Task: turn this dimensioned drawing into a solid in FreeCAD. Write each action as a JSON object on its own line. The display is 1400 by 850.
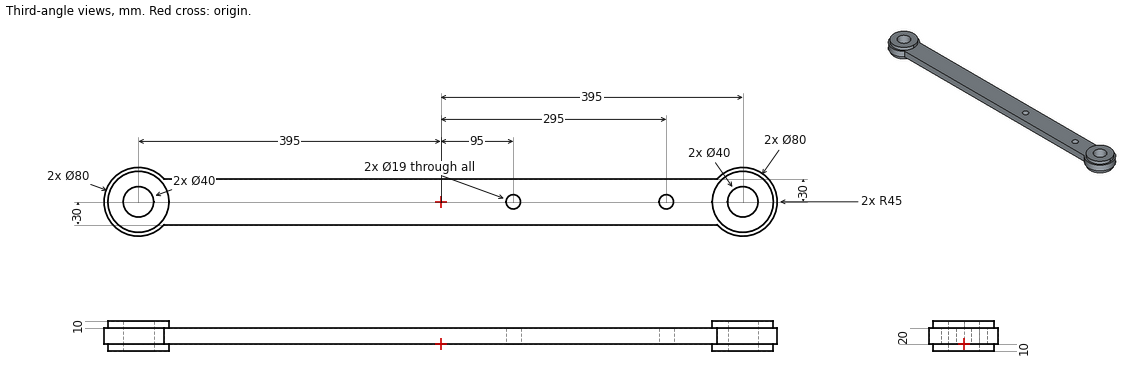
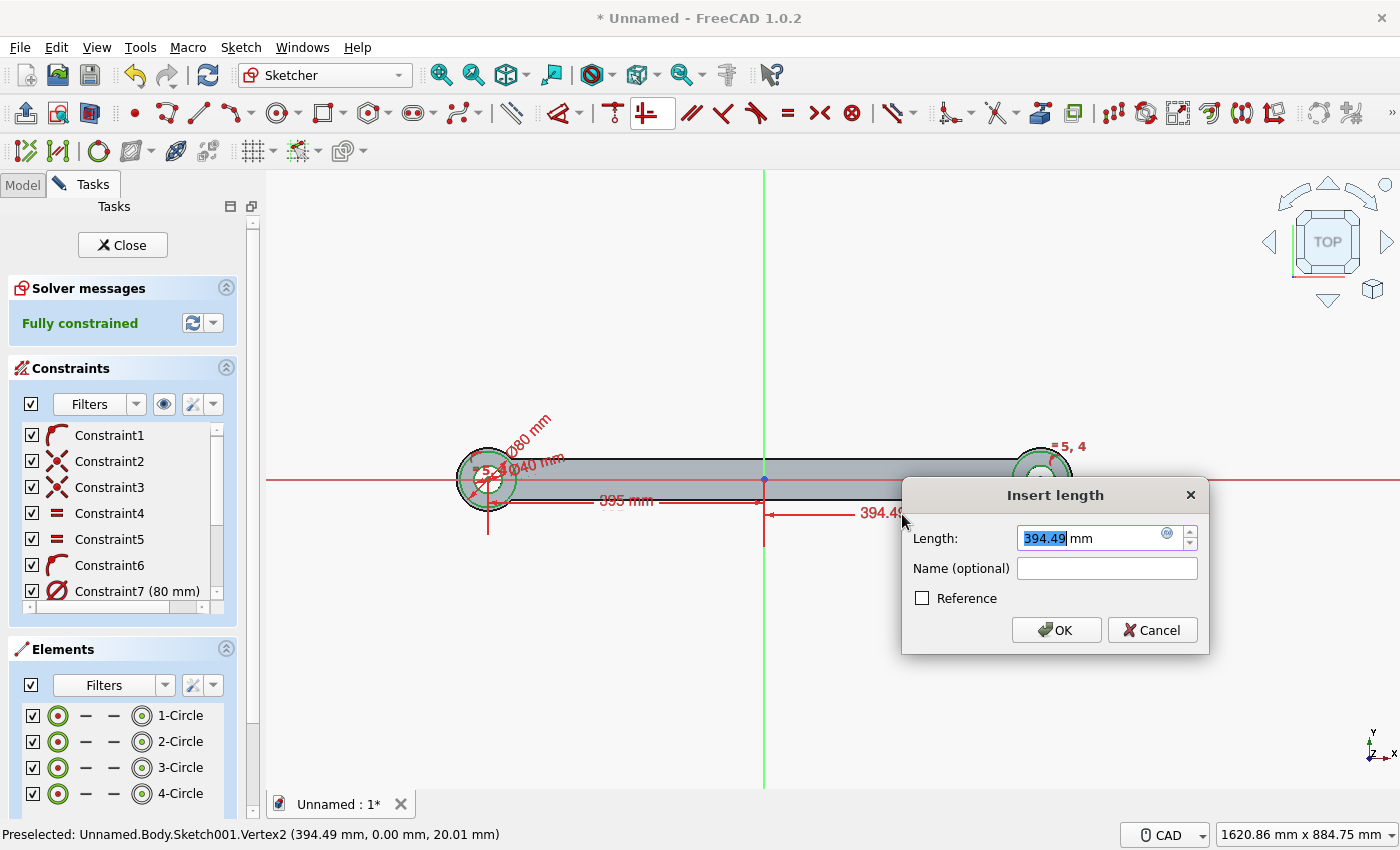
{"action": "type", "text": "395"}
{"action": "key", "text": "Return"}
{"action": "key", "text": "Escape"}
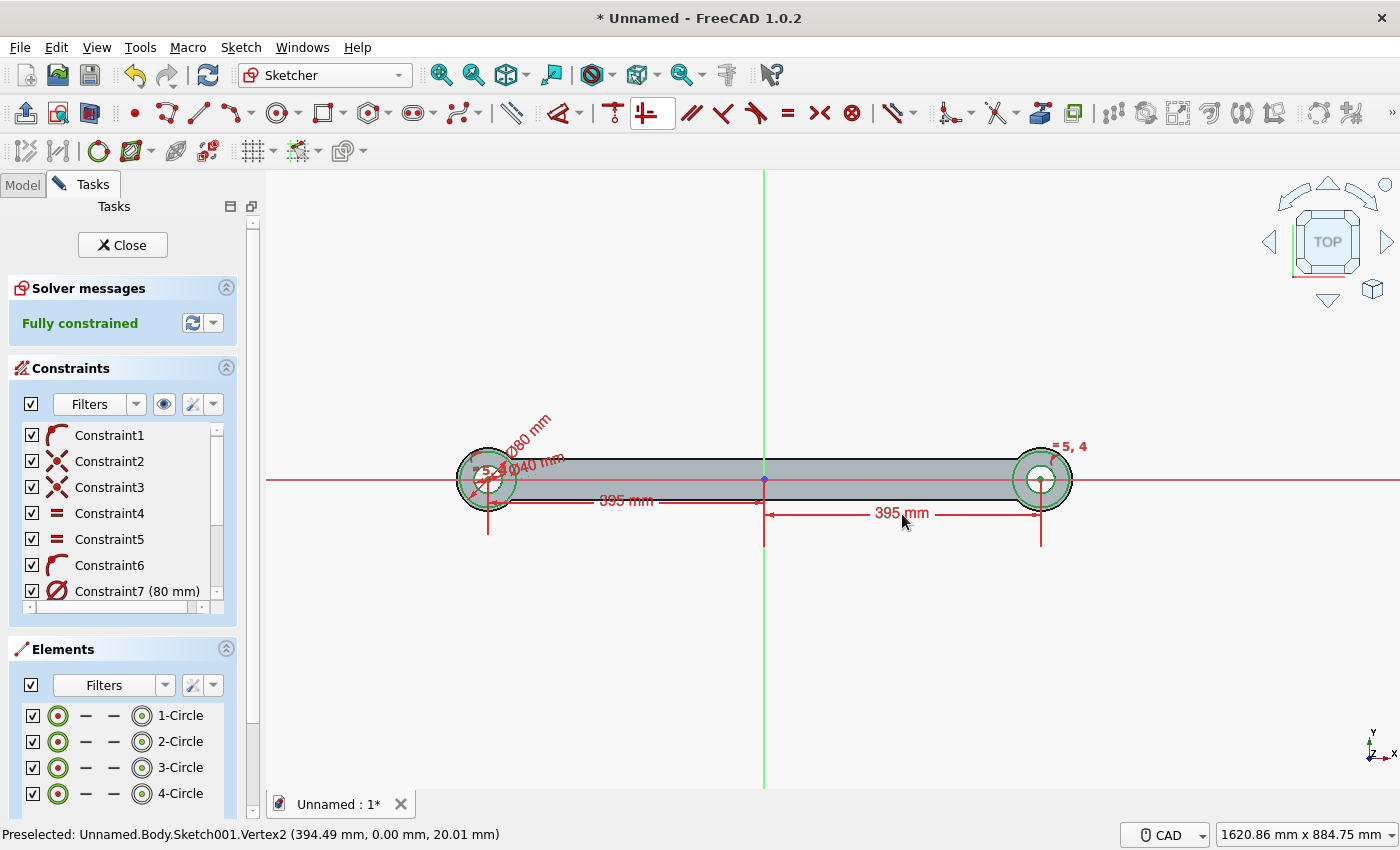
{"action": "left_click", "coordinate": [123, 245]}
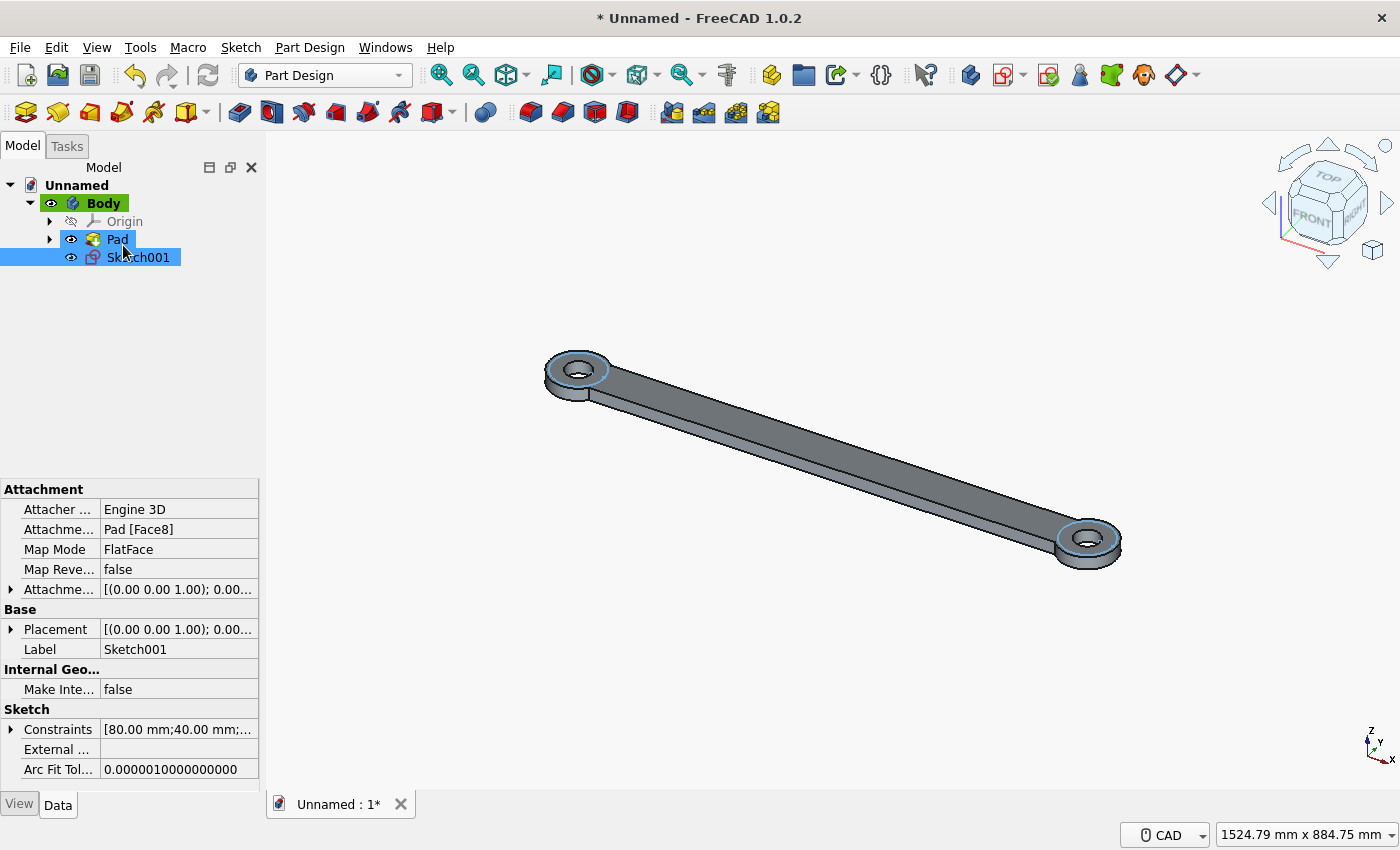
{"action": "left_click", "coordinate": [26, 112]}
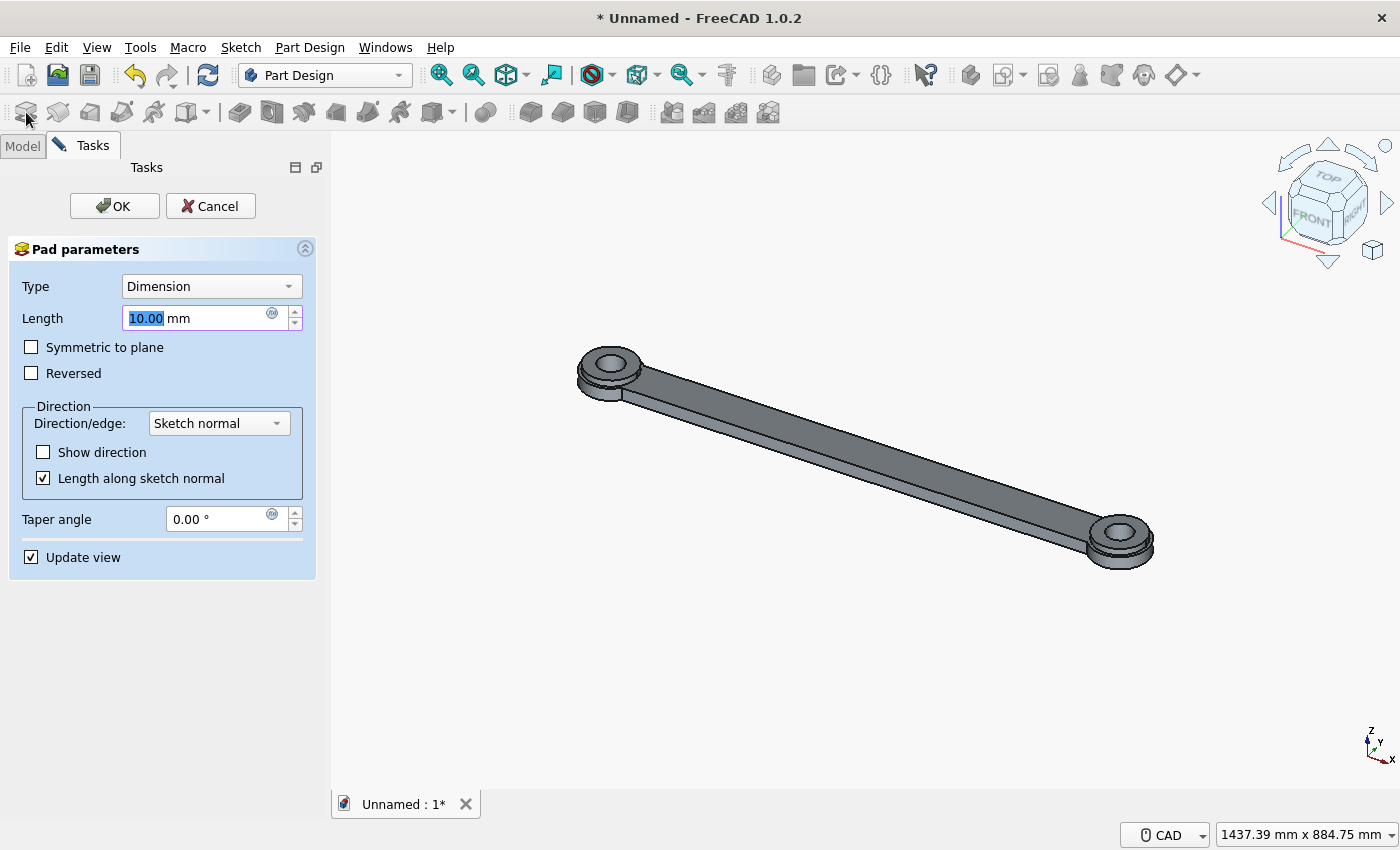
{"action": "type", "text": "10"}
{"action": "key", "text": "Tab"}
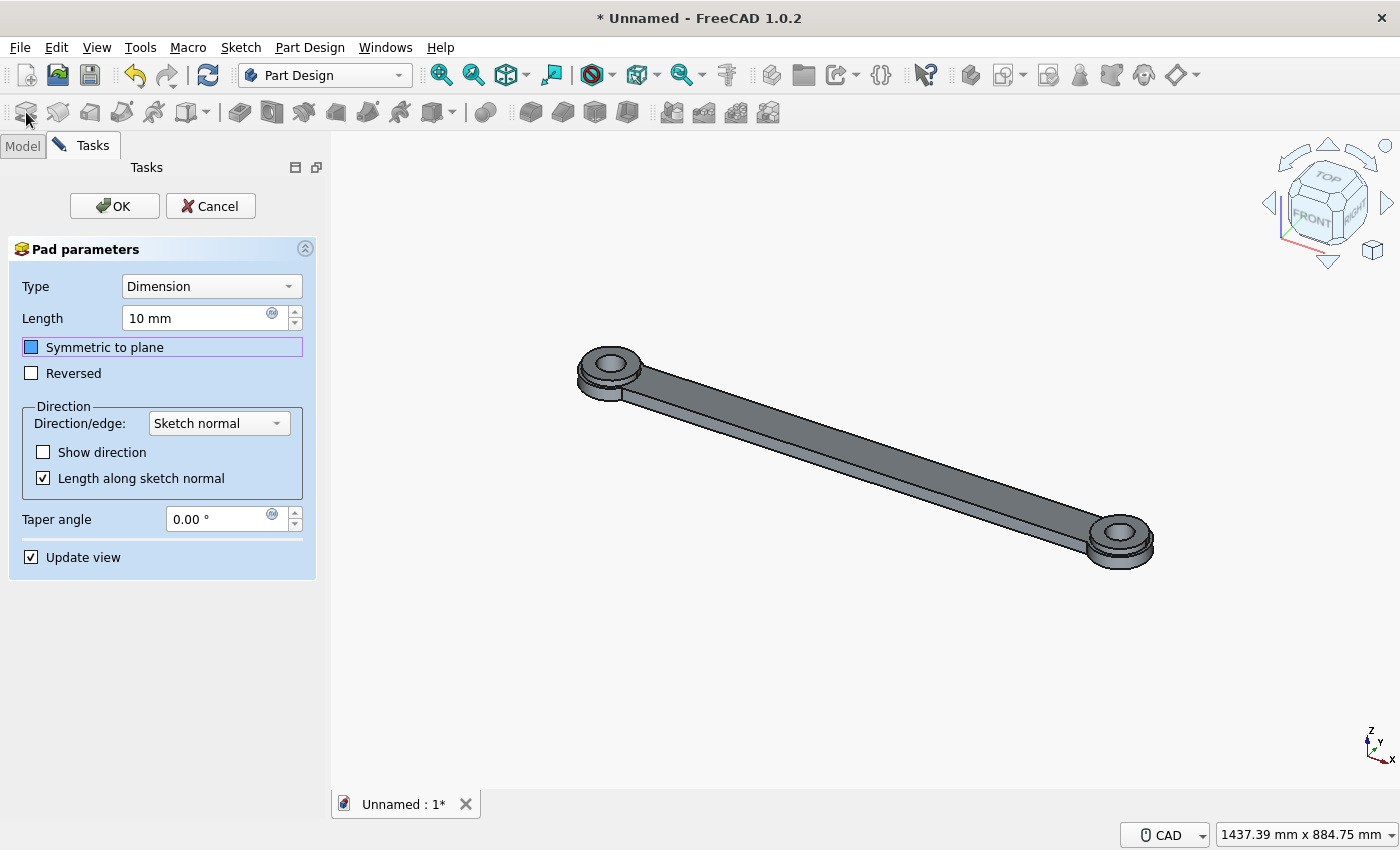
{"action": "left_click", "coordinate": [115, 206]}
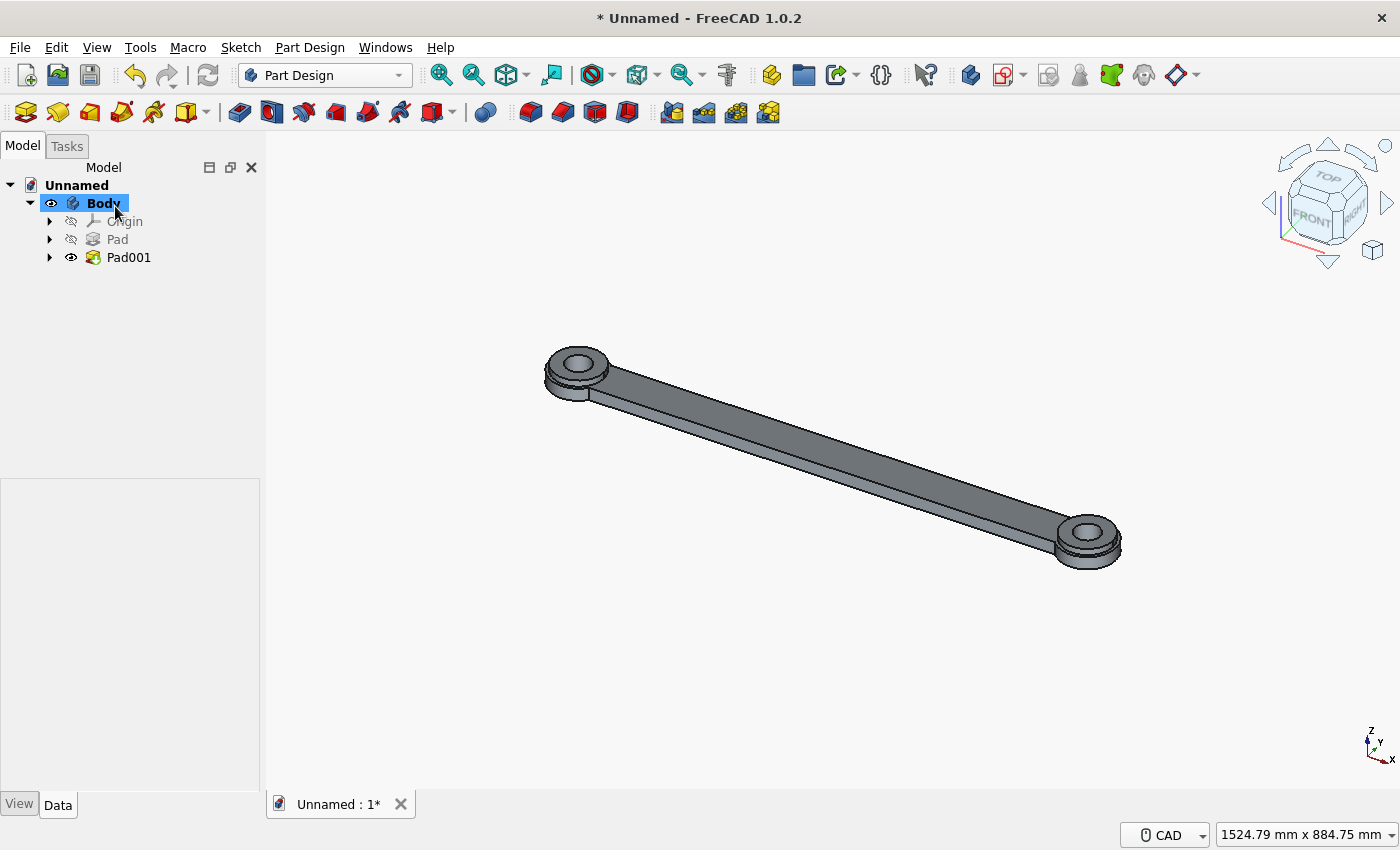
{"action": "left_click", "coordinate": [50, 221]}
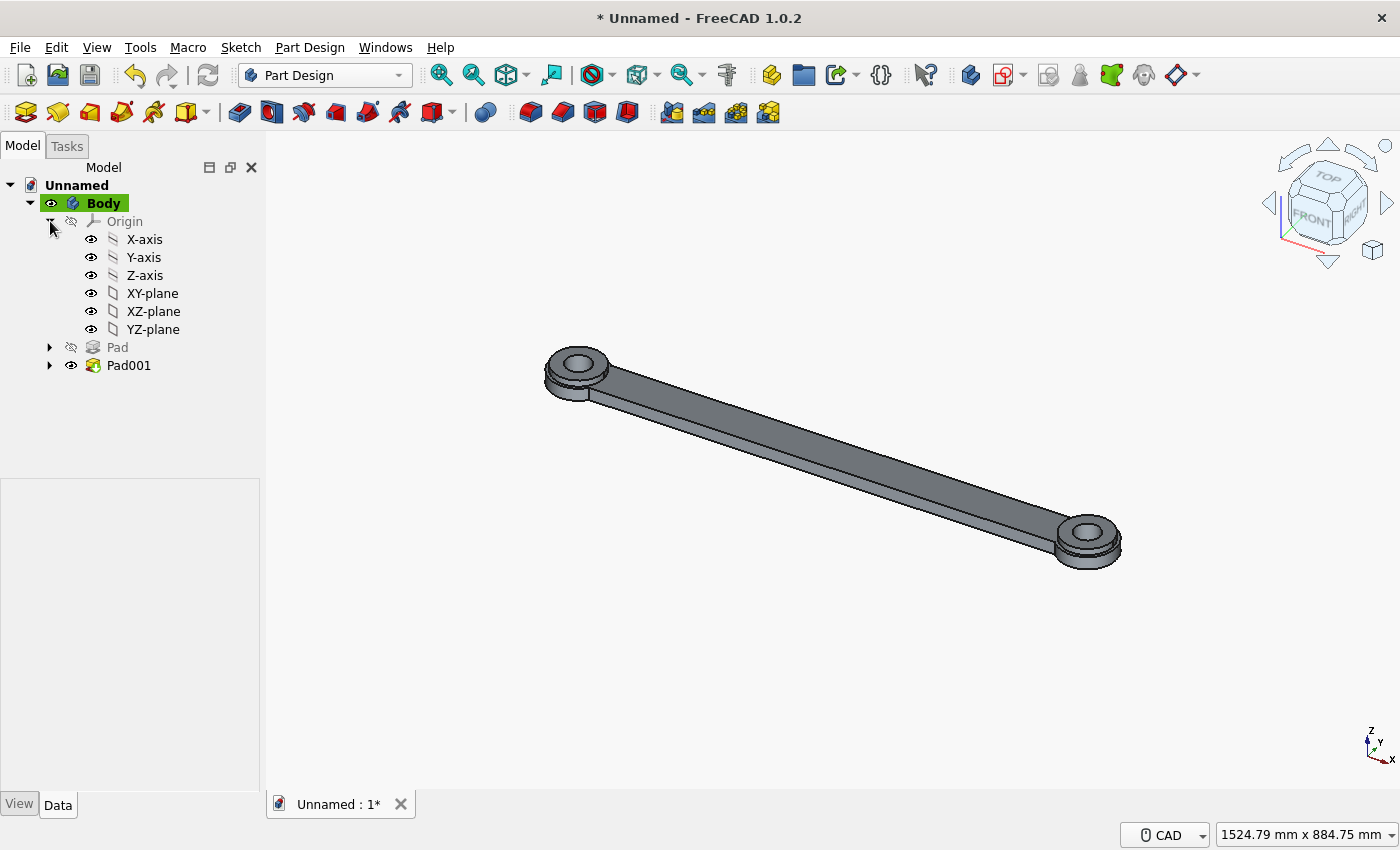
{"action": "left_click", "coordinate": [136, 293]}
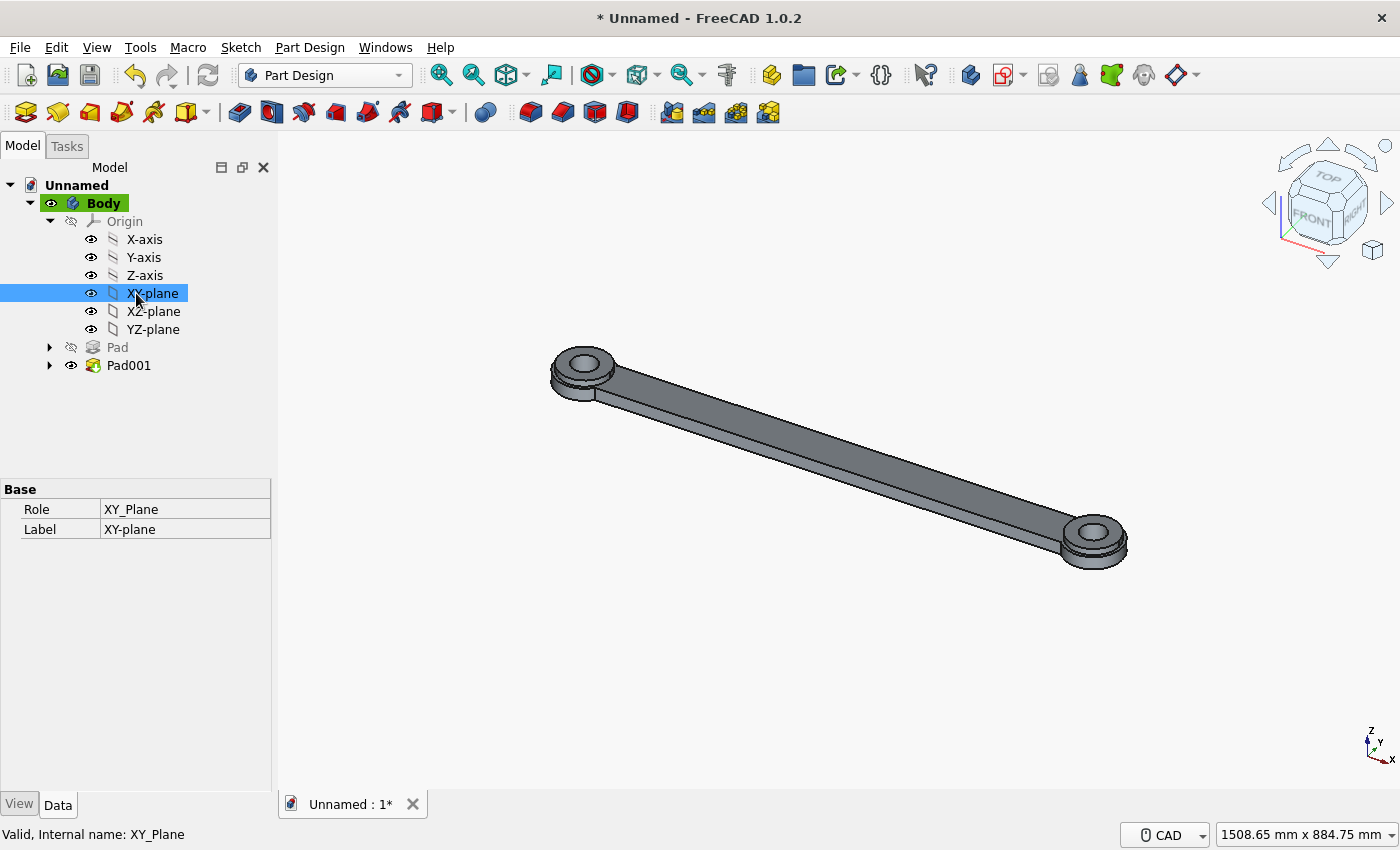
{"action": "left_click", "coordinate": [1176, 76]}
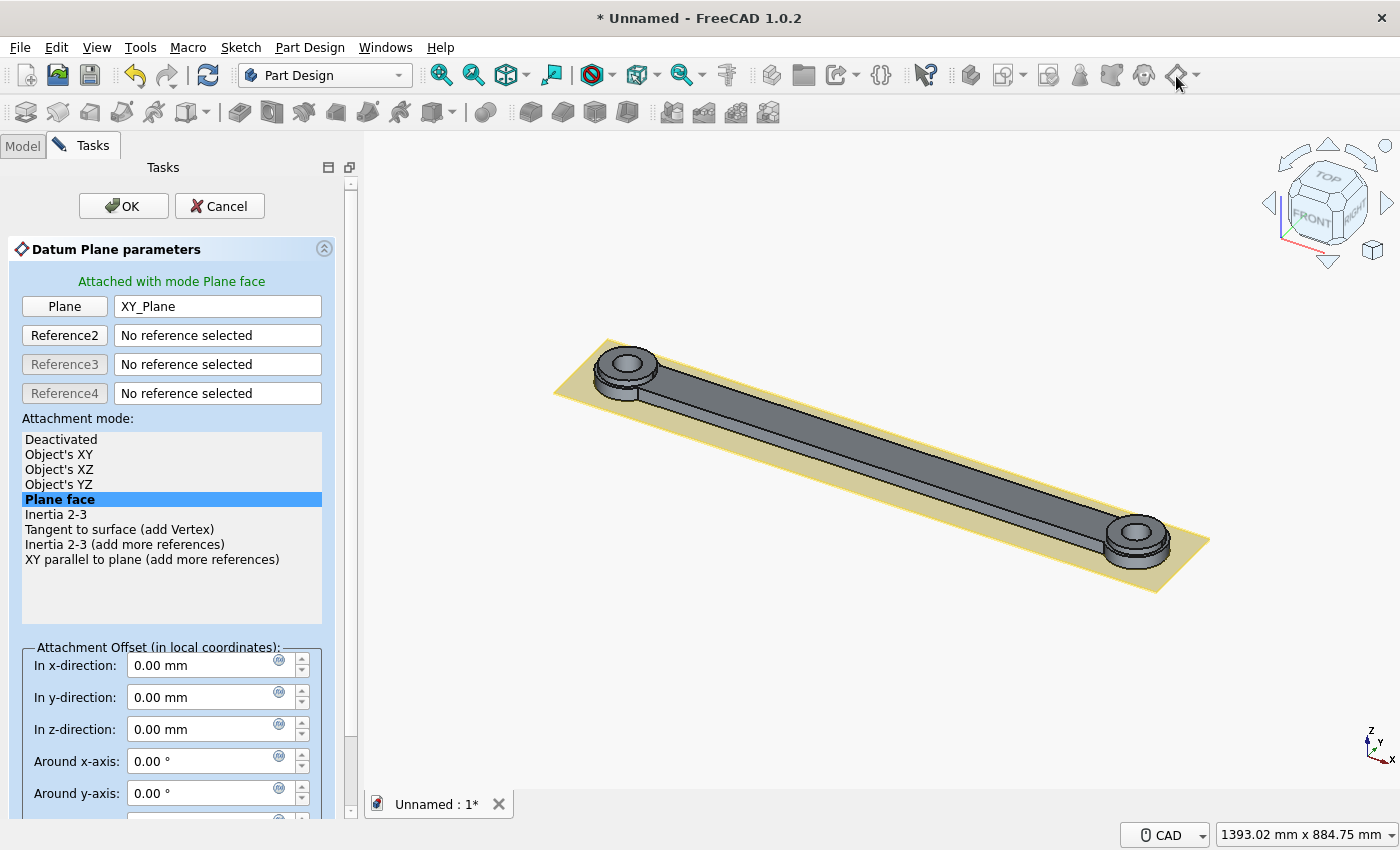
{"action": "triple_click", "coordinate": [210, 729]}